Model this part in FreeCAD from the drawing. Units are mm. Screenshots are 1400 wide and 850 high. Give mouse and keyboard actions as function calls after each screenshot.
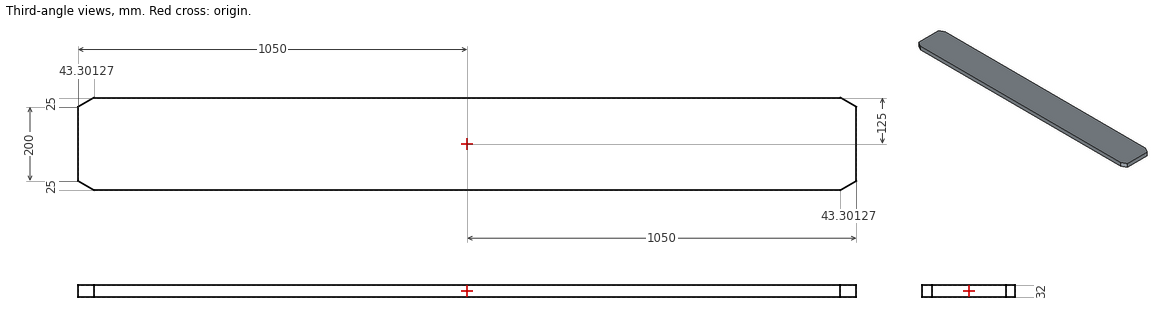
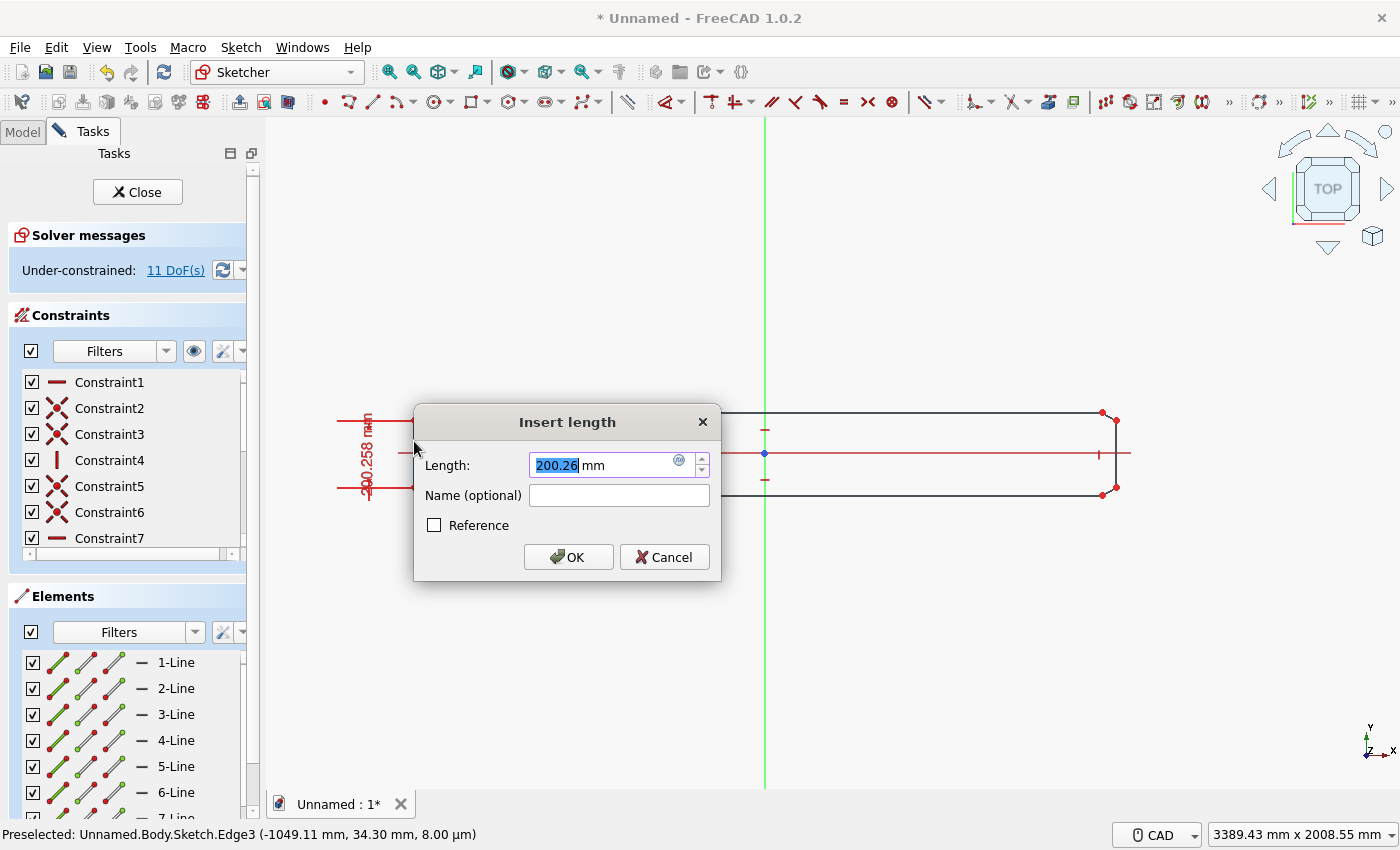
text(200)
key(Return)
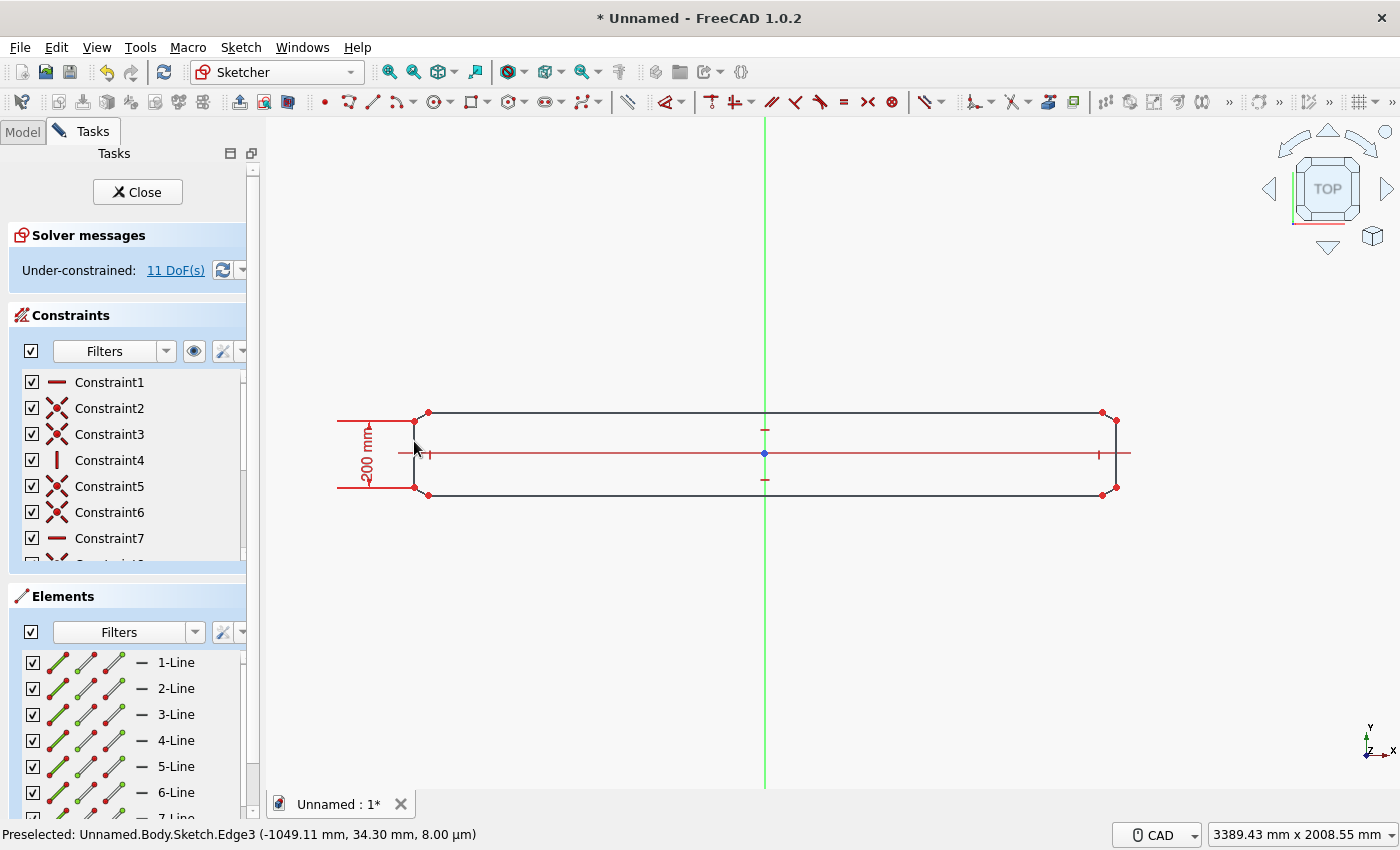
click(1116, 468)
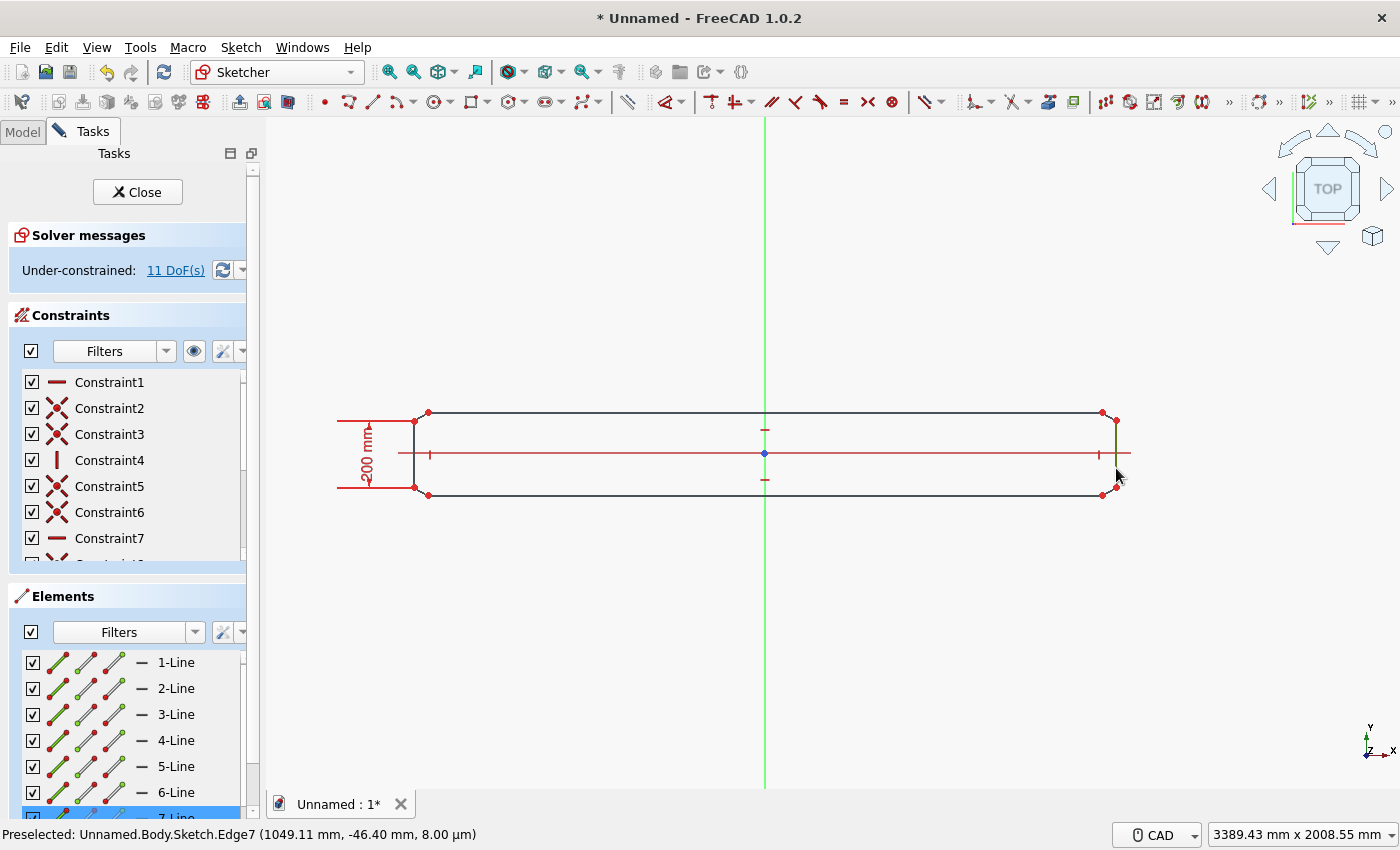
click(684, 102)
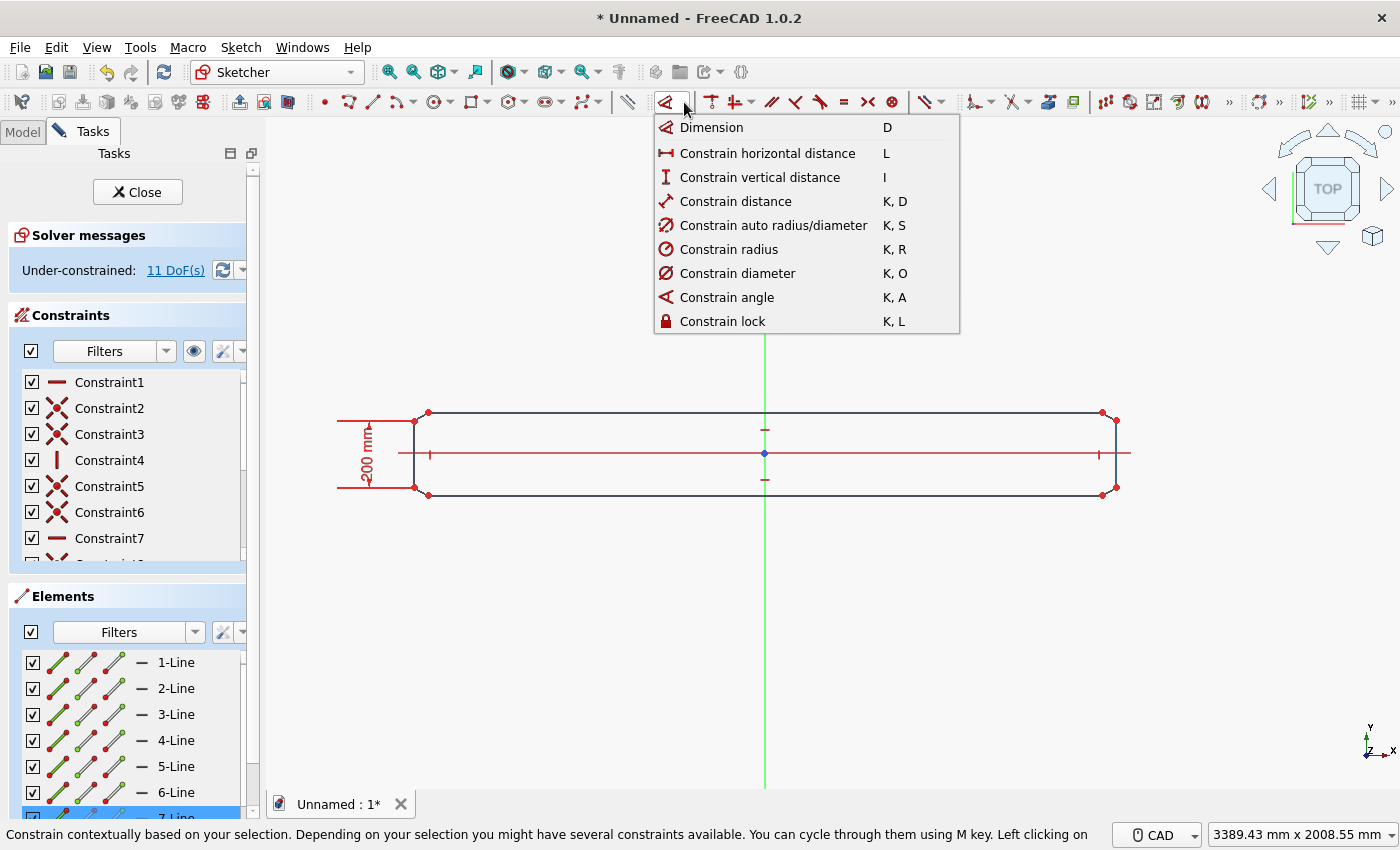
click(807, 177)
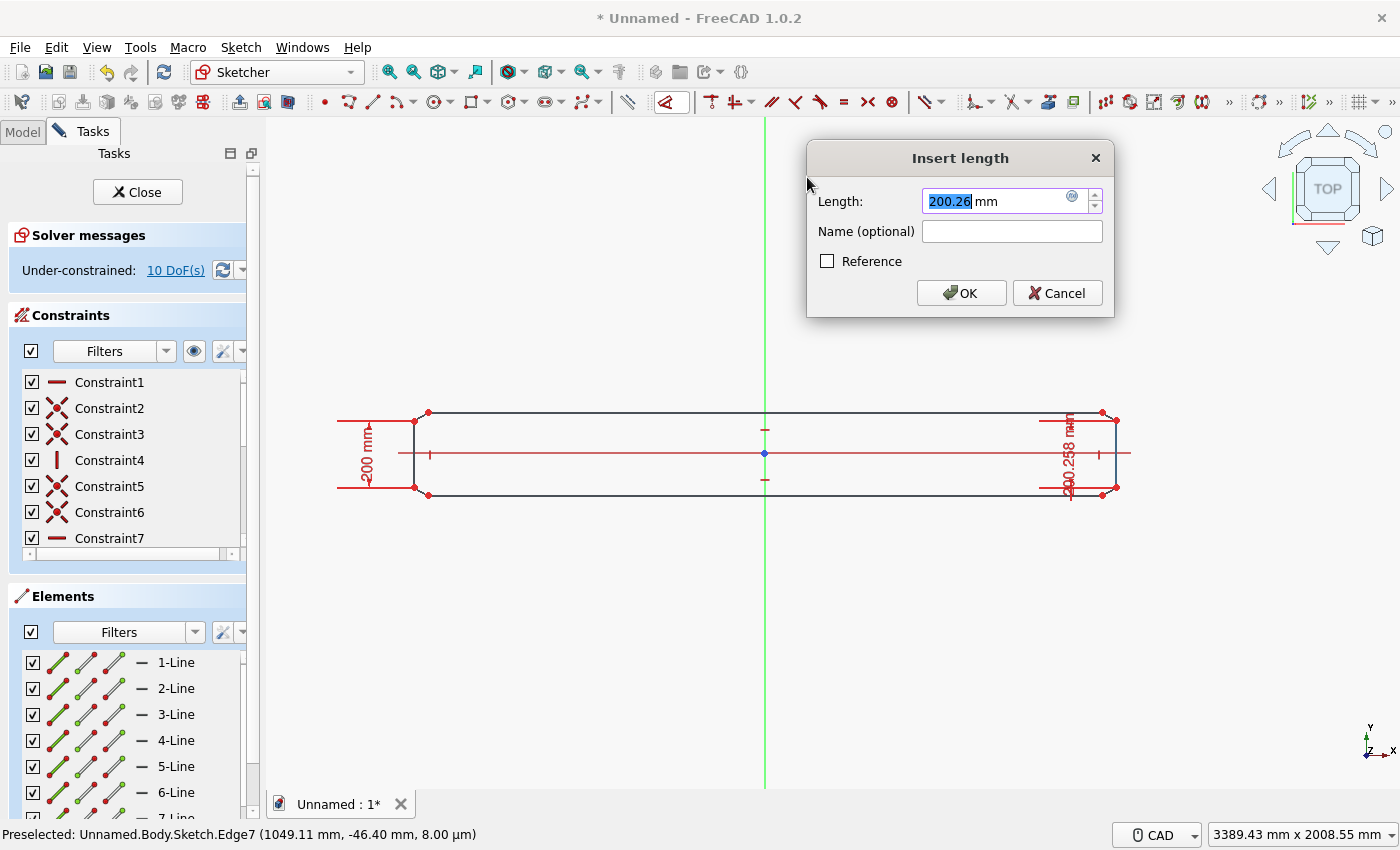
text(200)
key(Return)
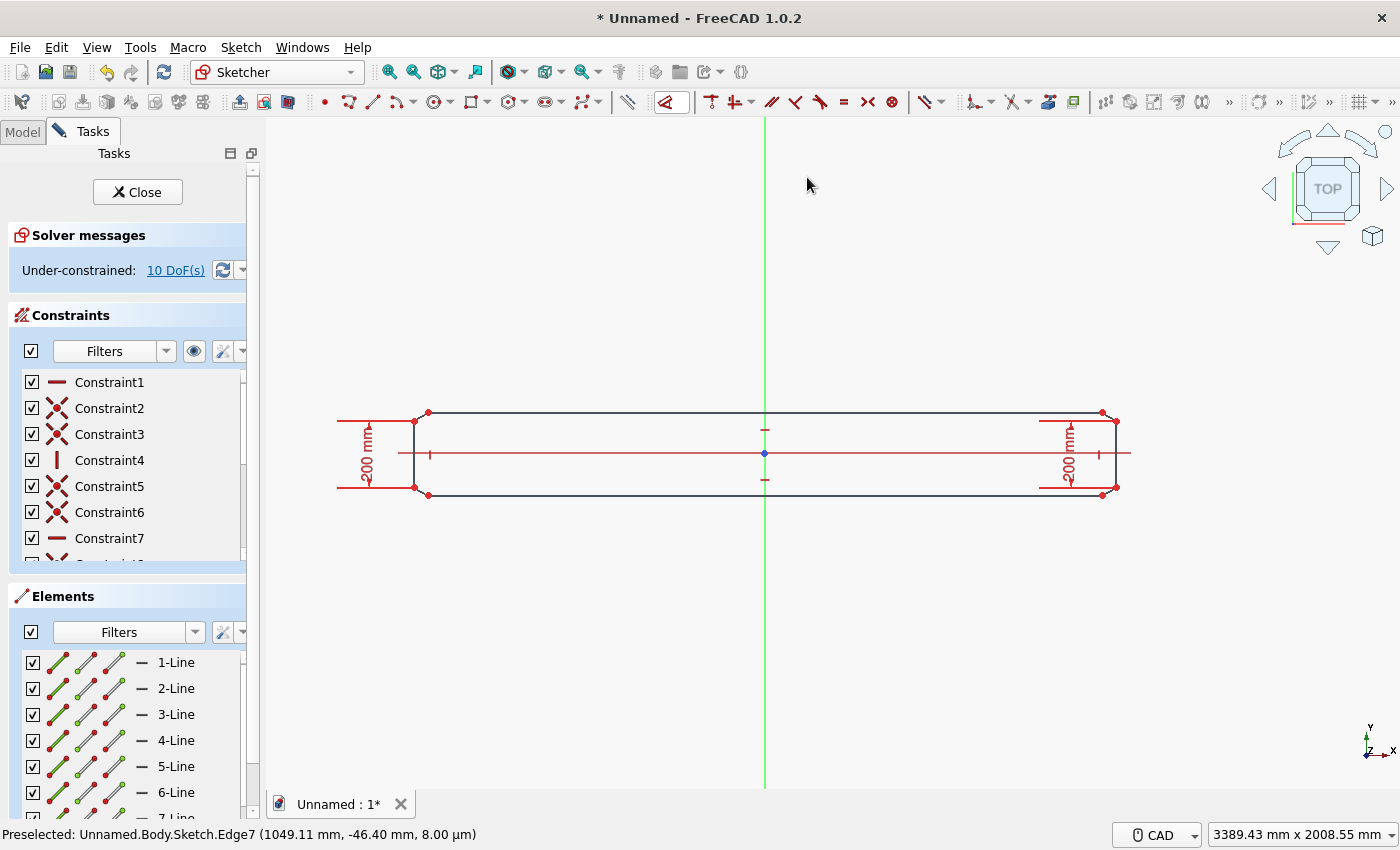
scroll(421, 417, up, 8)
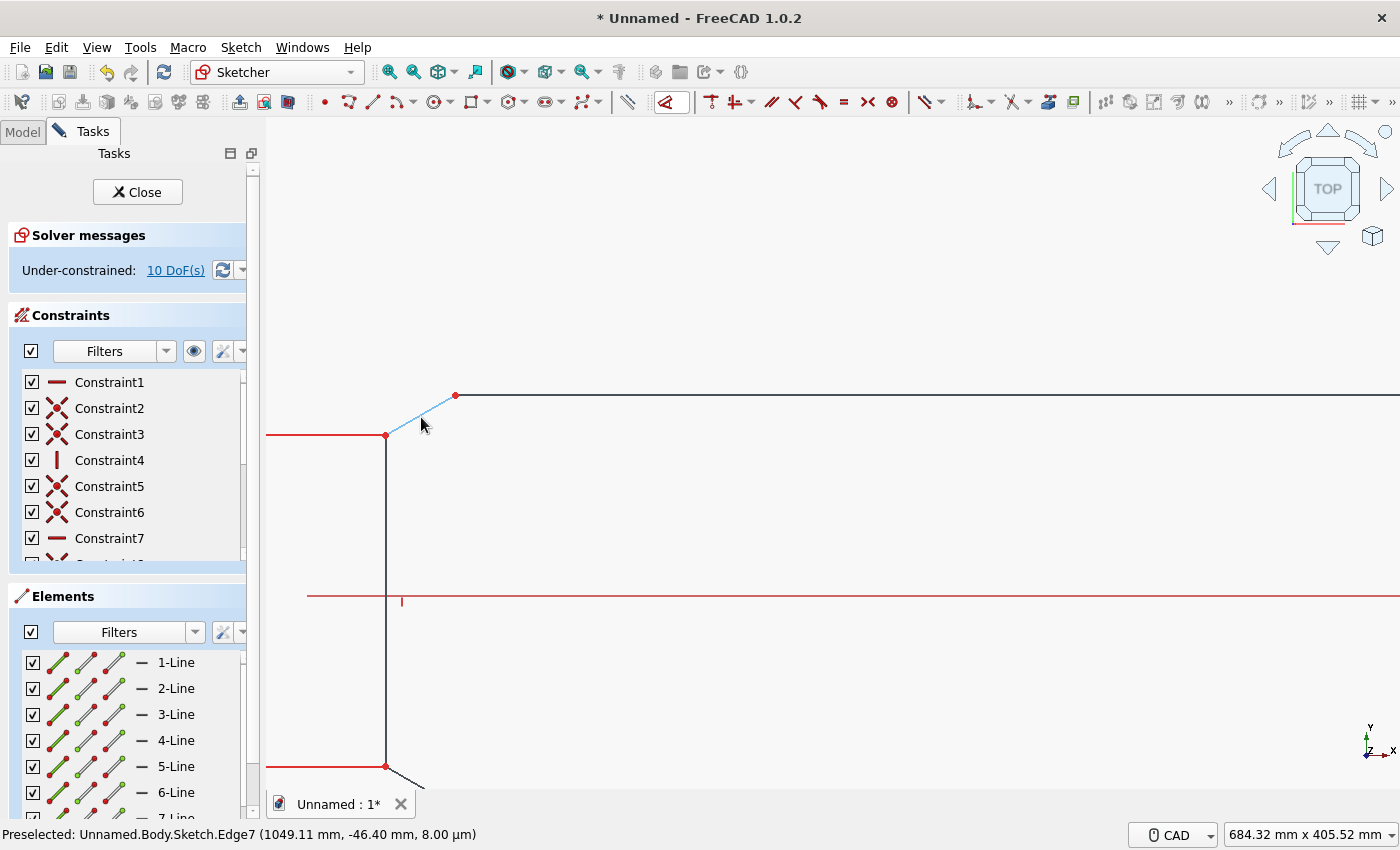
click(420, 415)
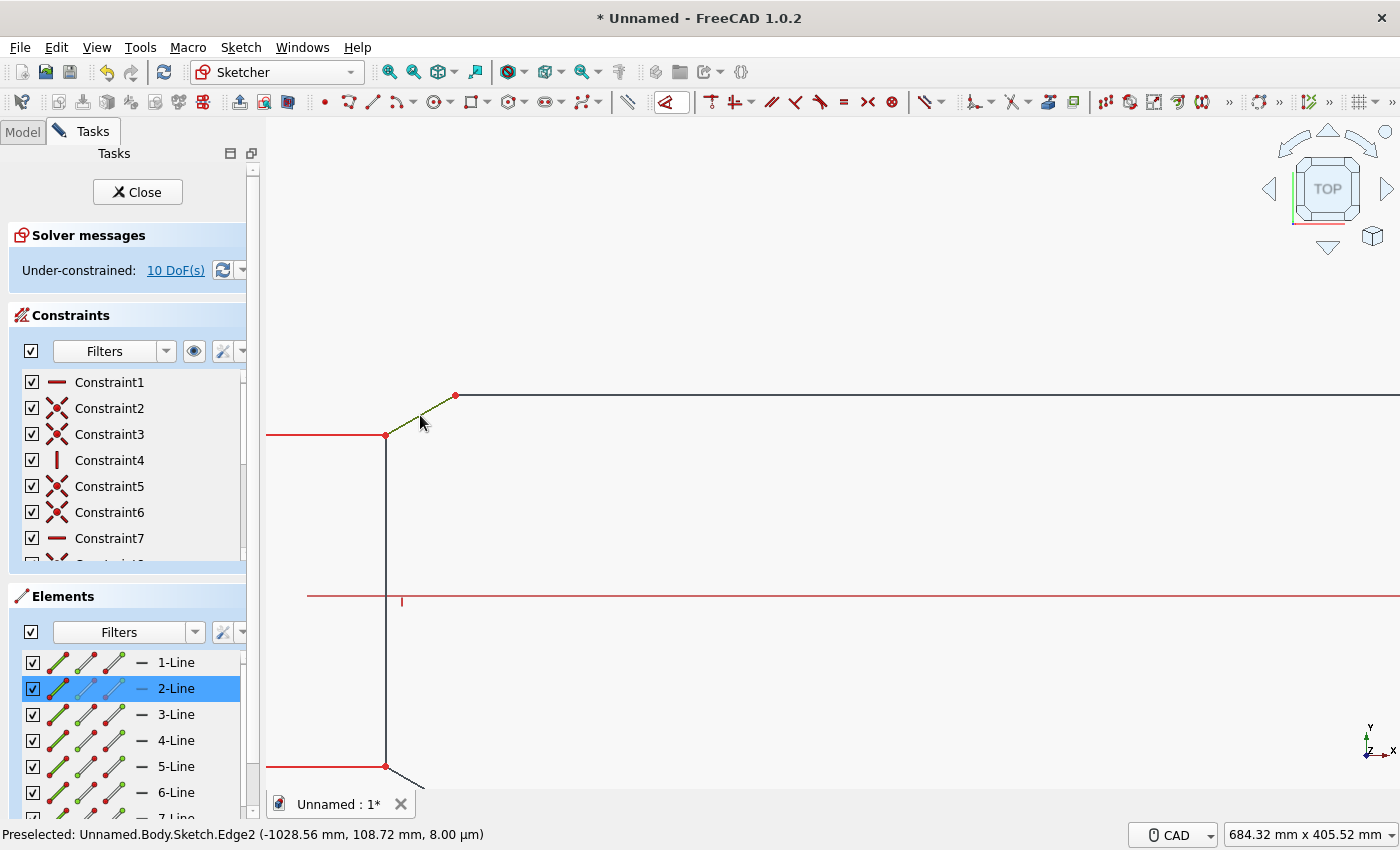
click(684, 102)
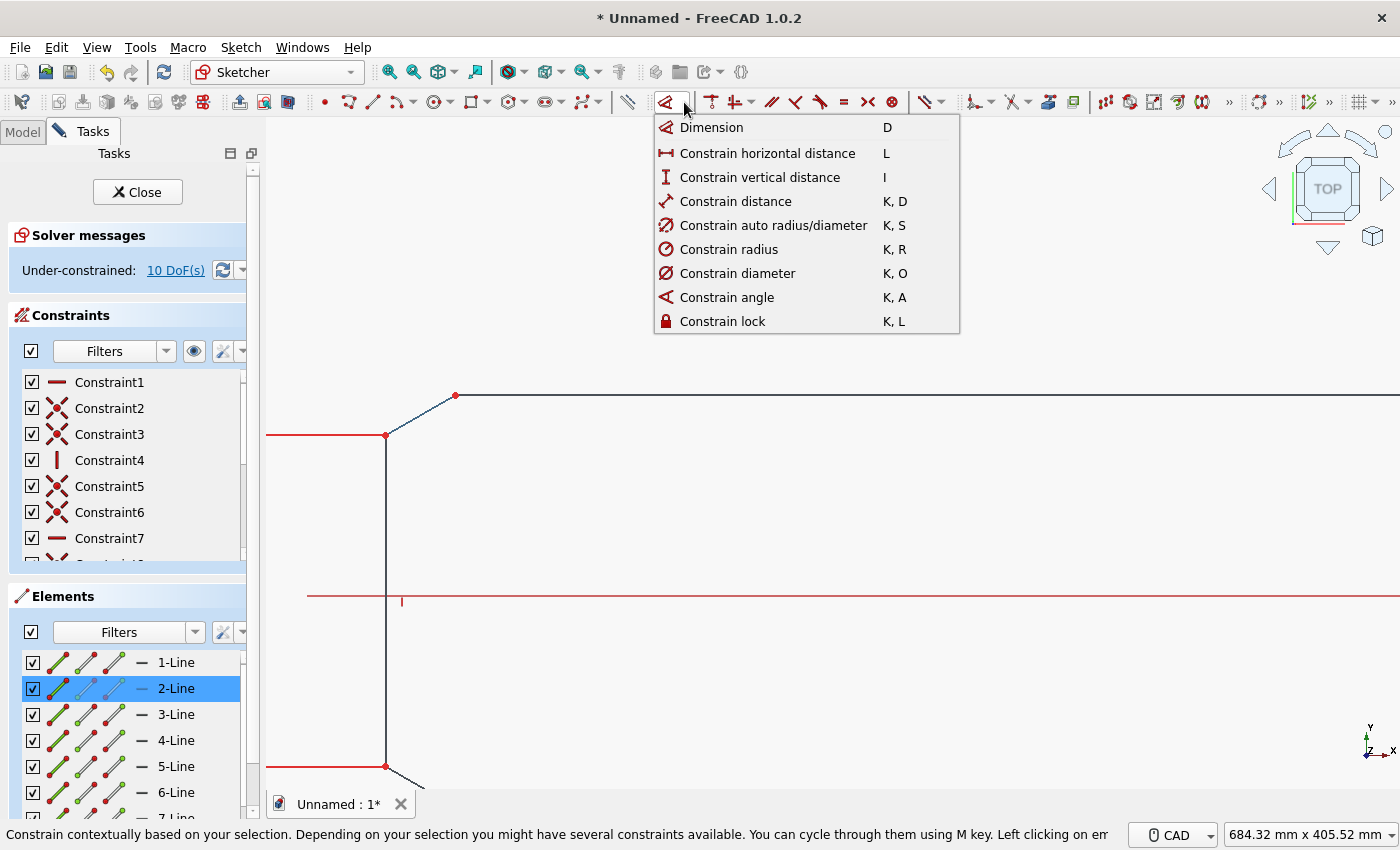
click(807, 177)